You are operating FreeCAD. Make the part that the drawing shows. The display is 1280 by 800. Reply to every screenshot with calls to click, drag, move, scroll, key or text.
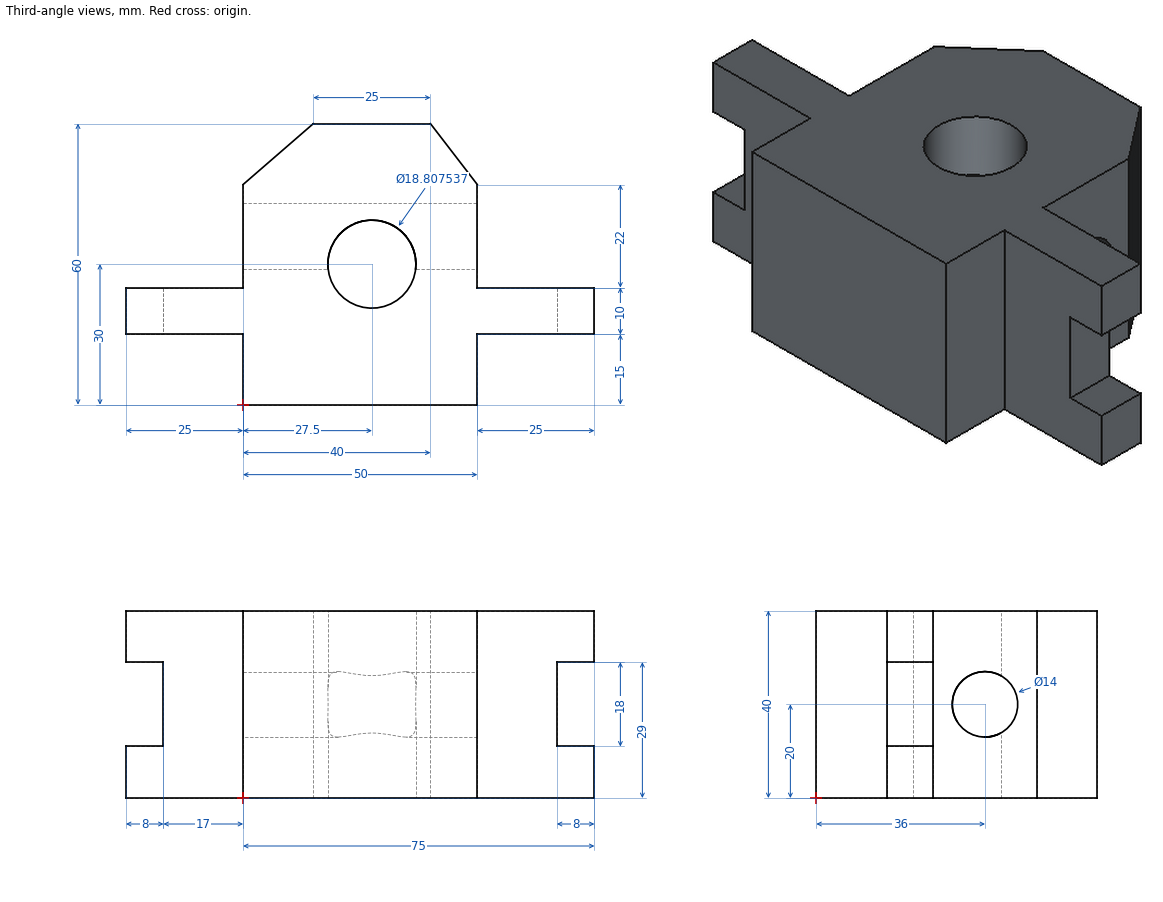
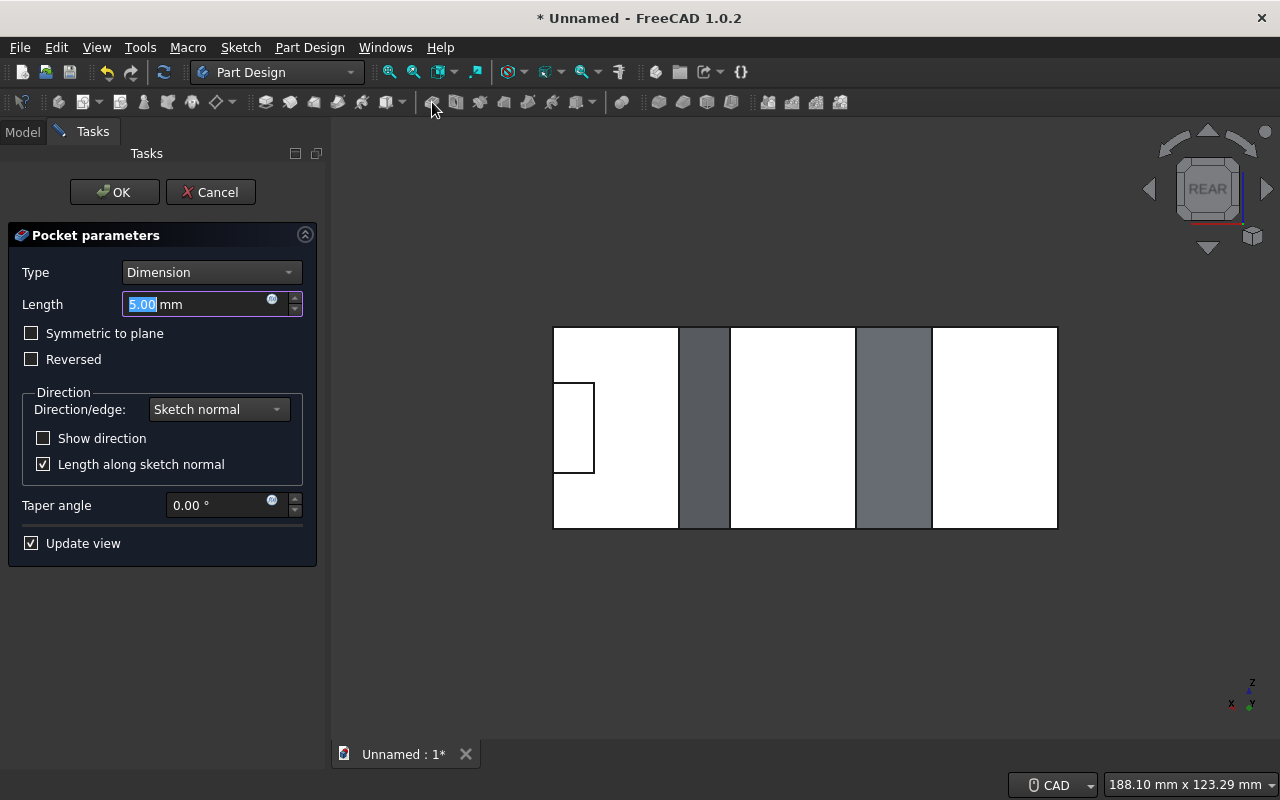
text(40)
key(Tab)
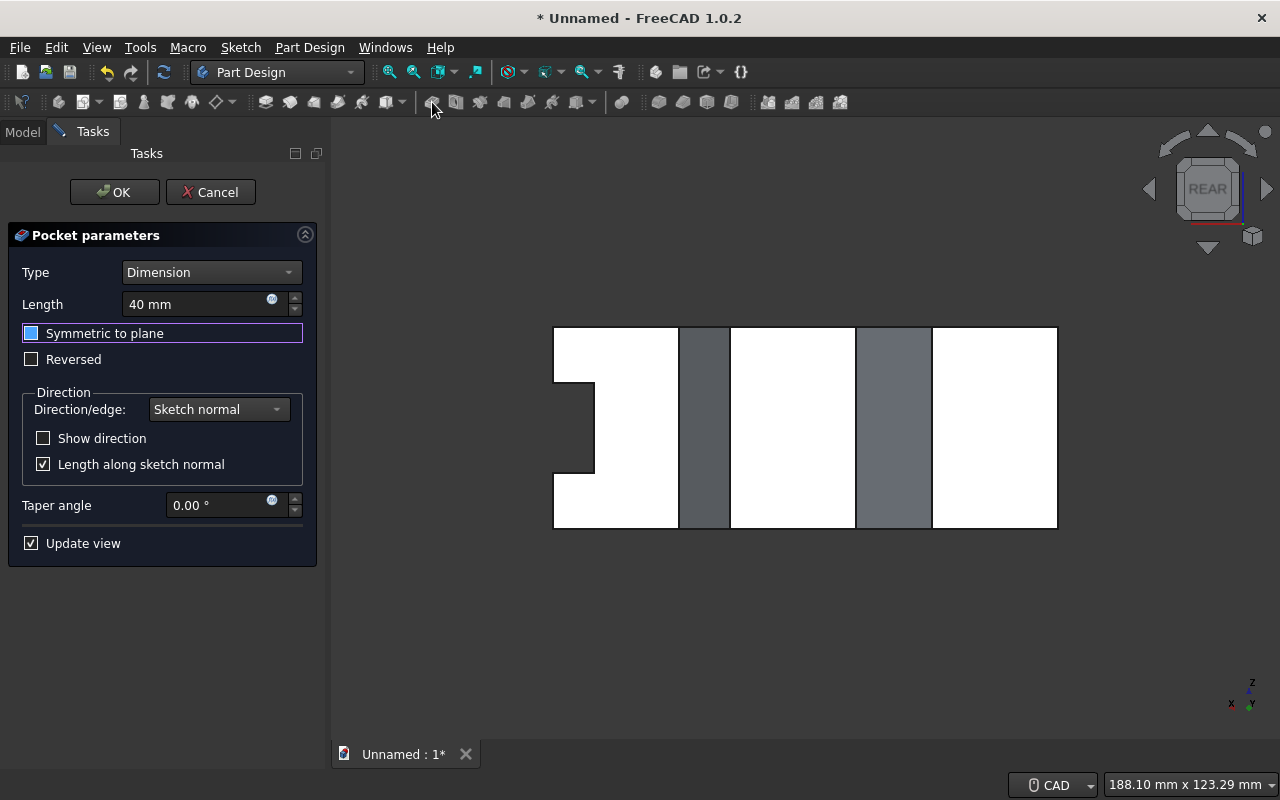
click(115, 192)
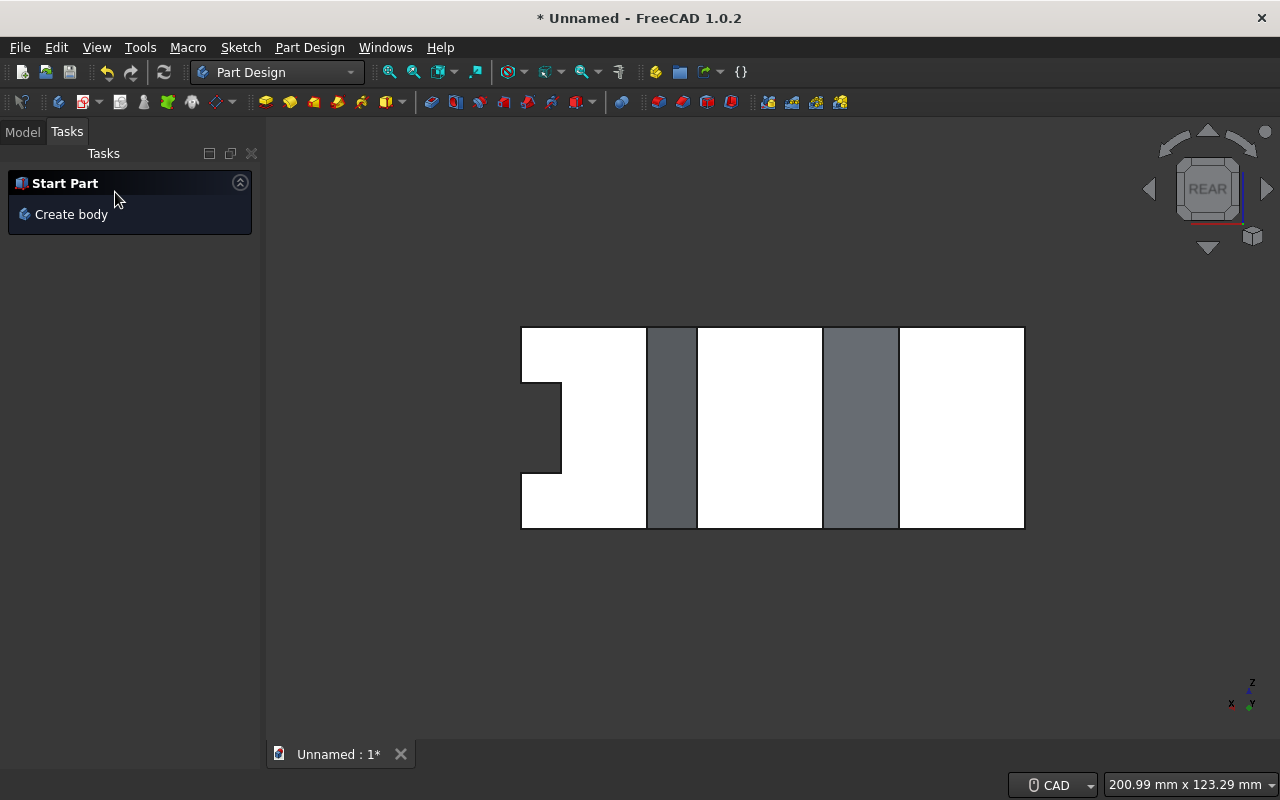
click(962, 398)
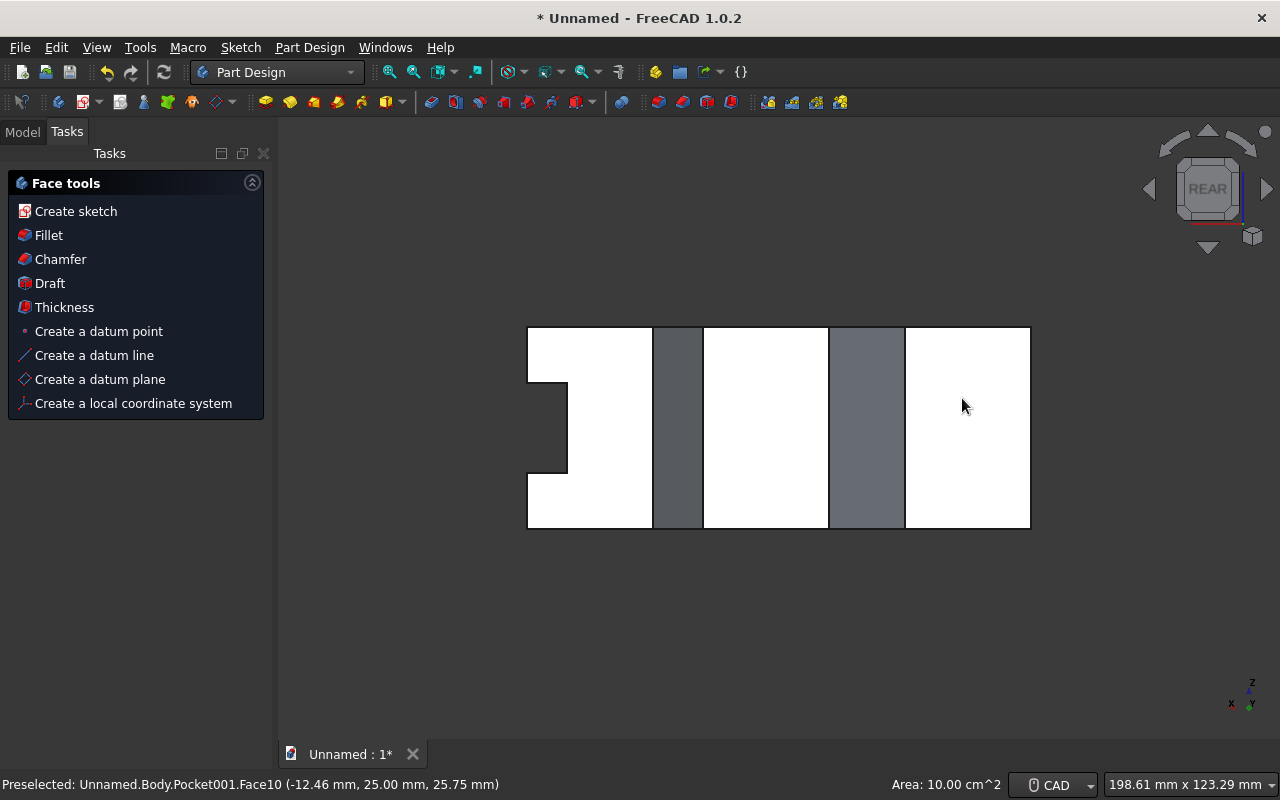
click(84, 102)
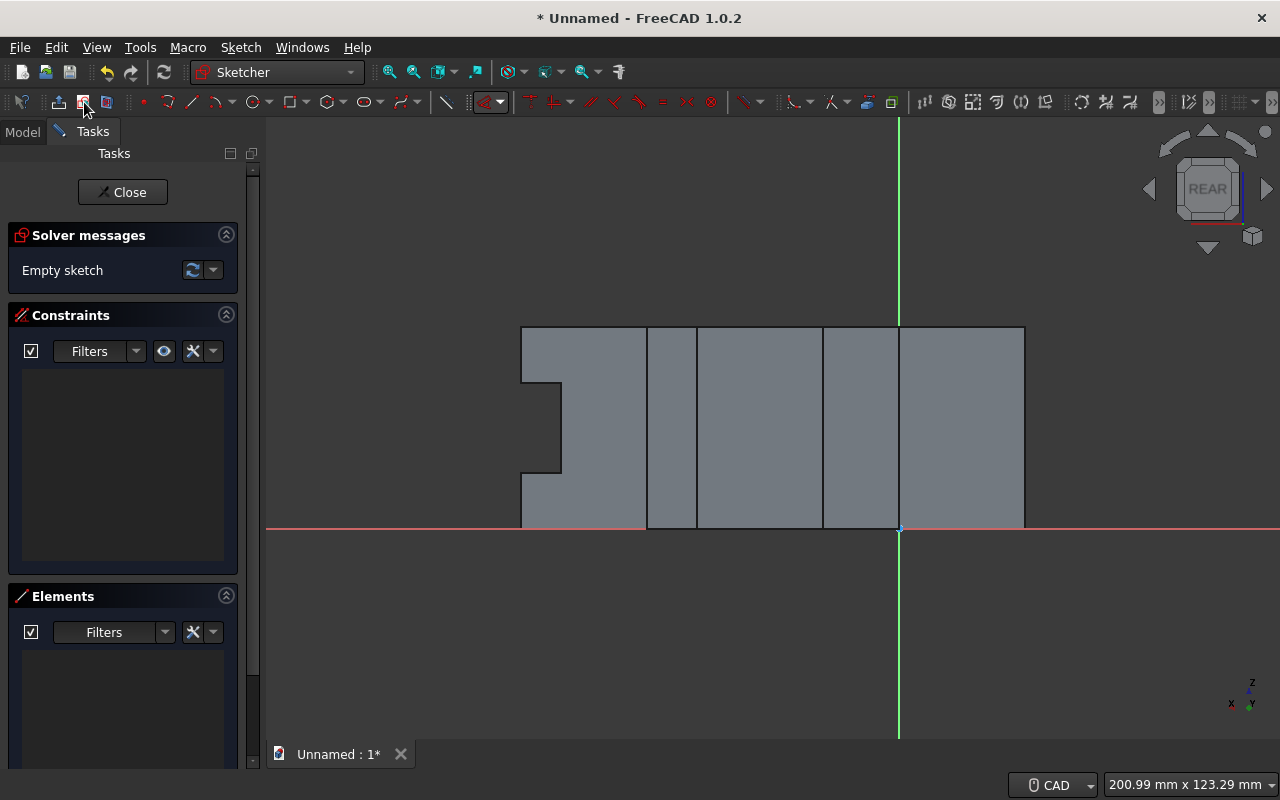
key(q)
key(s)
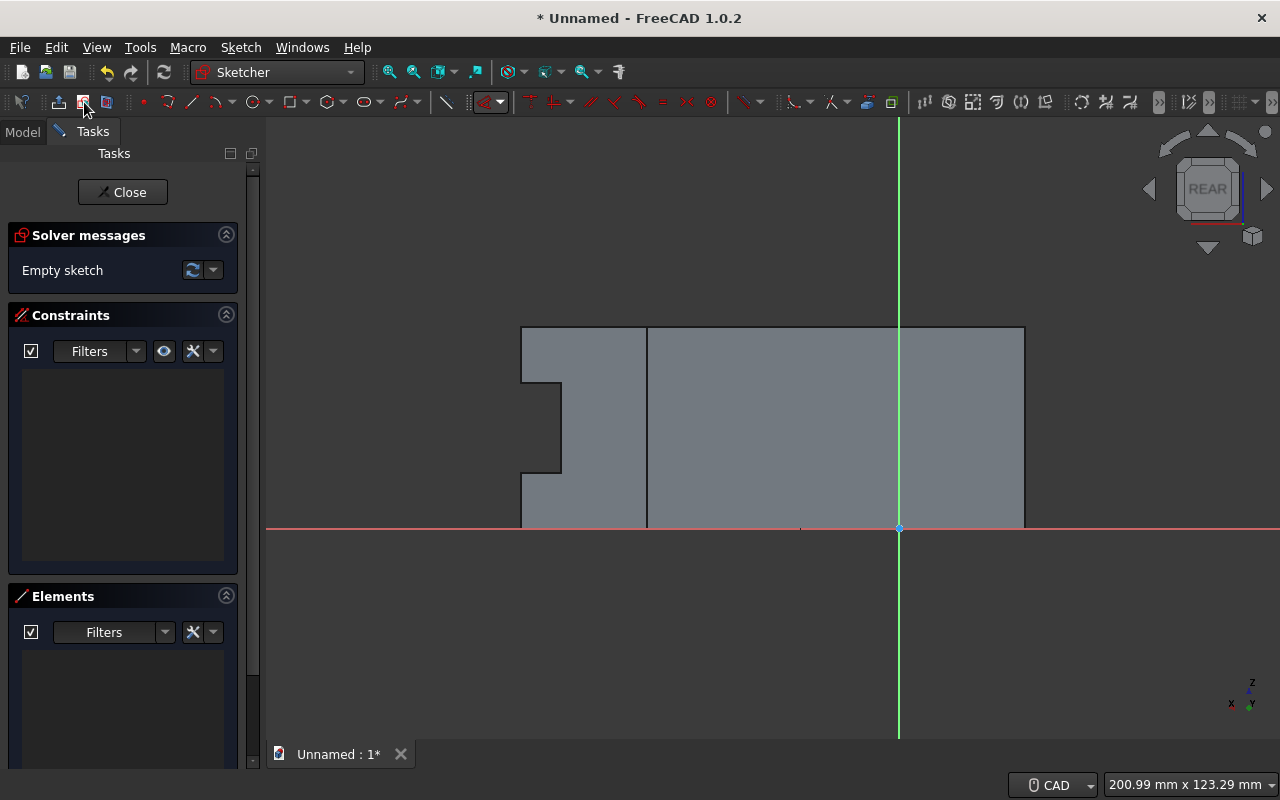
scroll(1112, 472, up, 5)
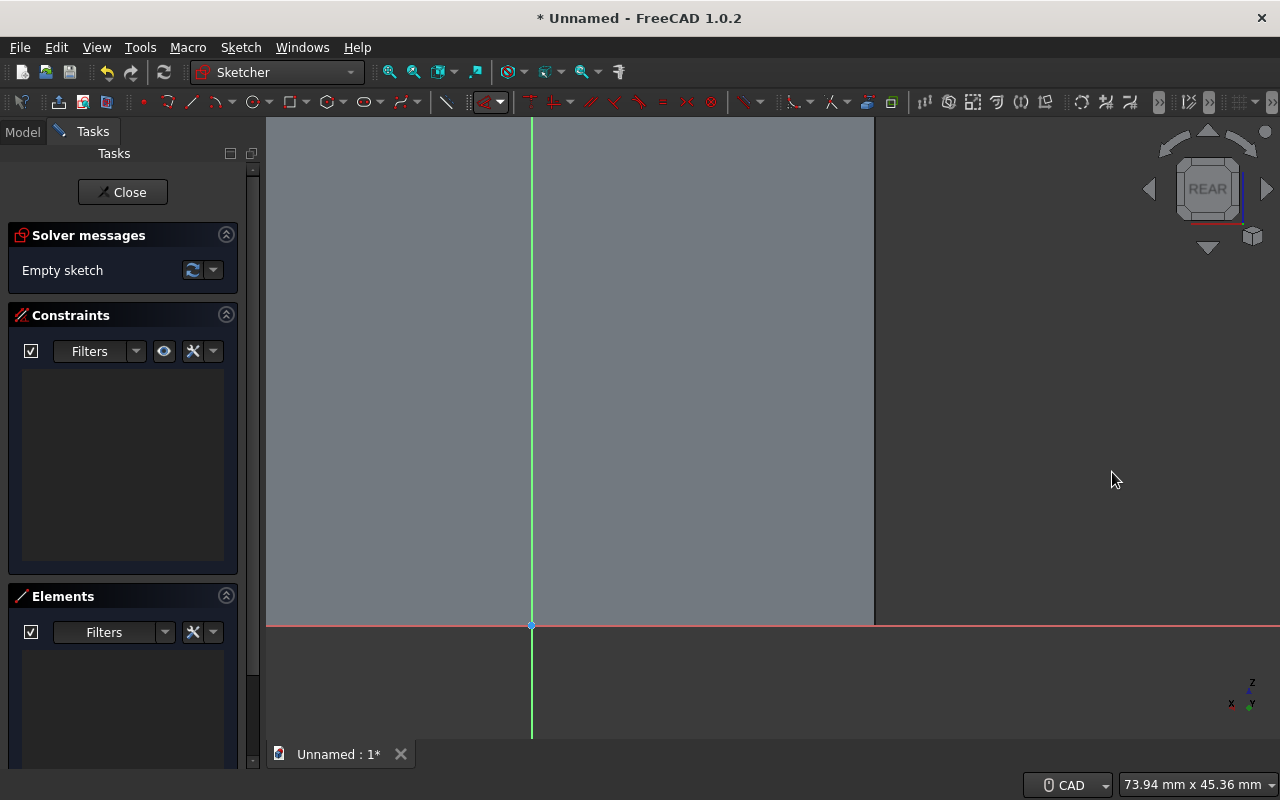
key(g)
key(r)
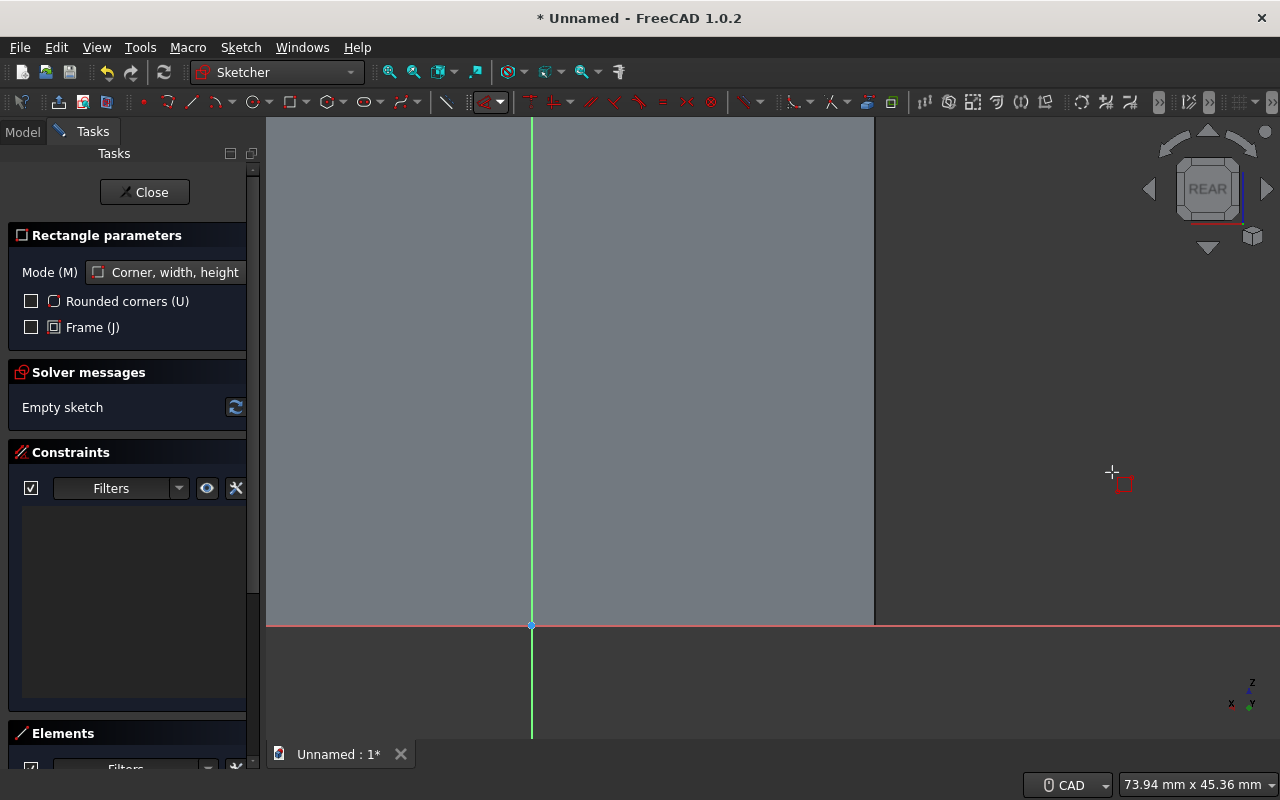
click(765, 228)
move(875, 475)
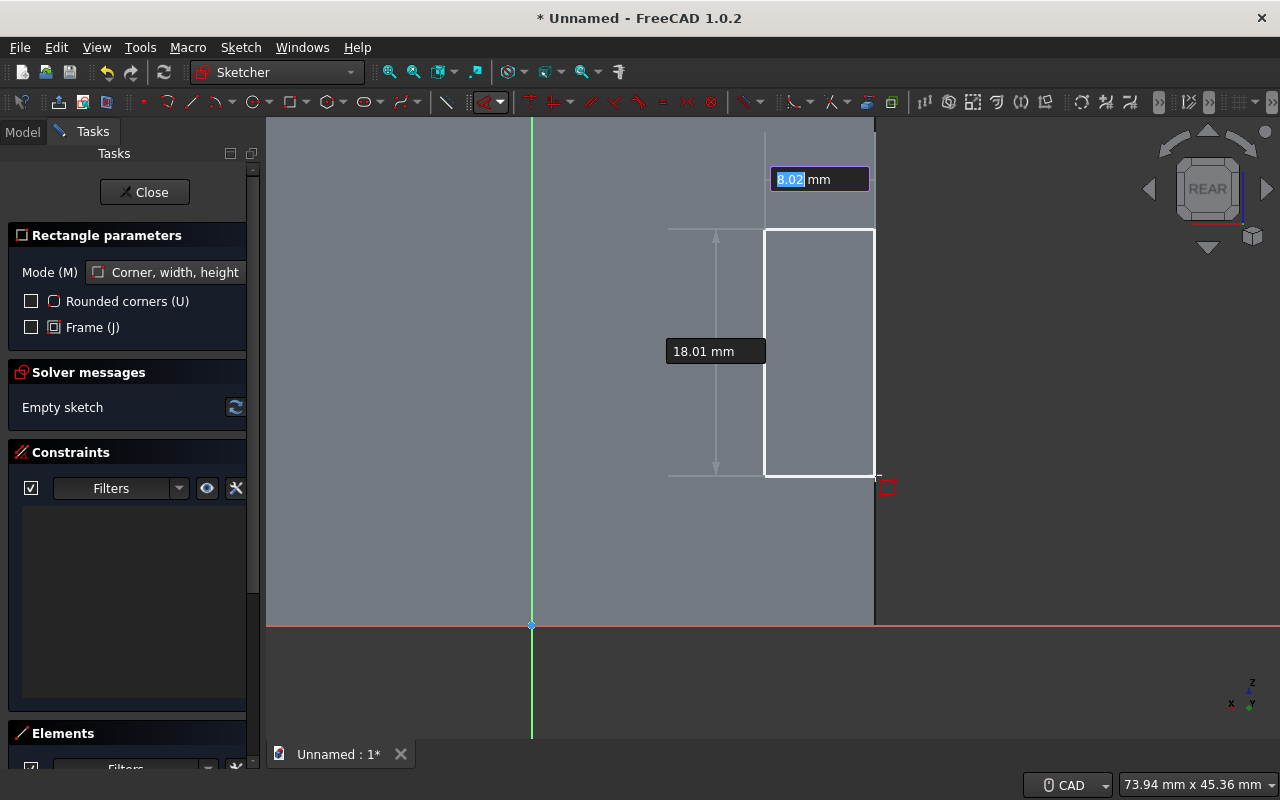
text(8)
key(Tab)
text(18)
key(Return)
key(Escape)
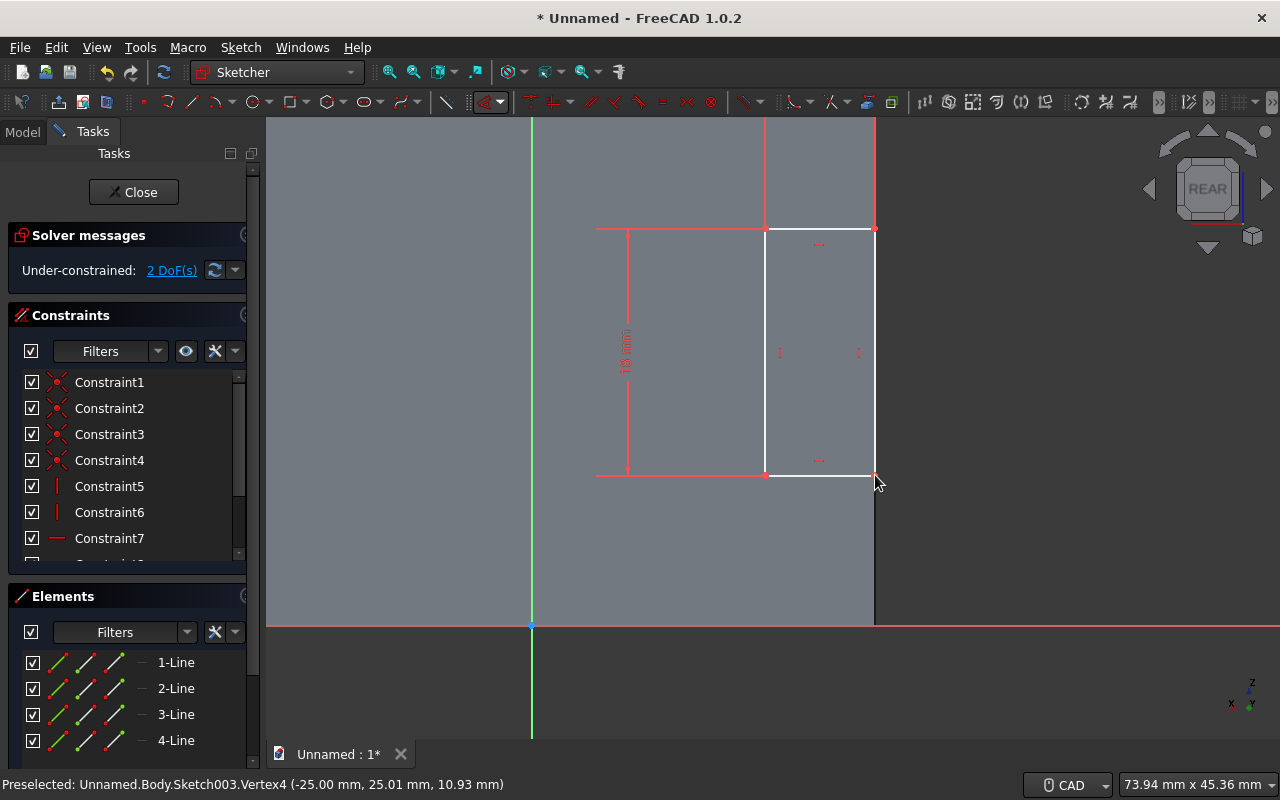
click(765, 229)